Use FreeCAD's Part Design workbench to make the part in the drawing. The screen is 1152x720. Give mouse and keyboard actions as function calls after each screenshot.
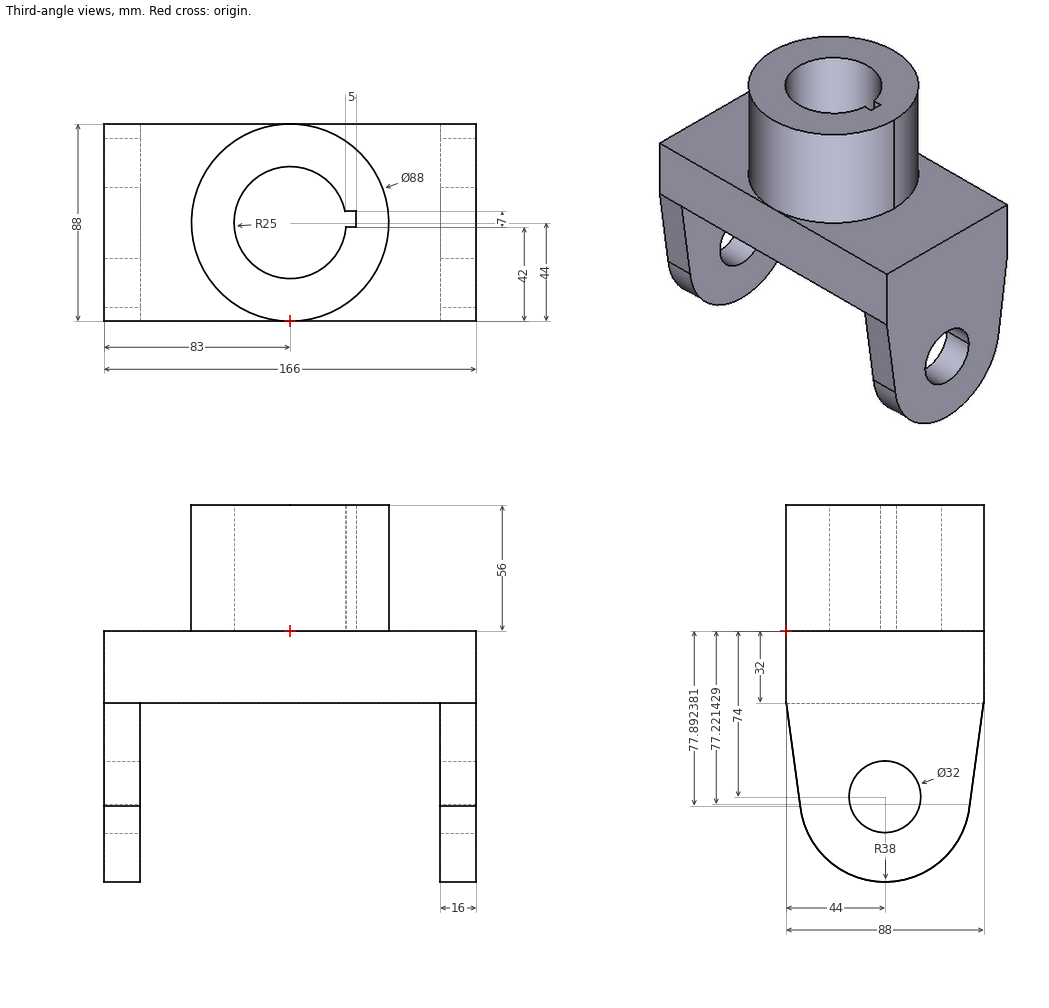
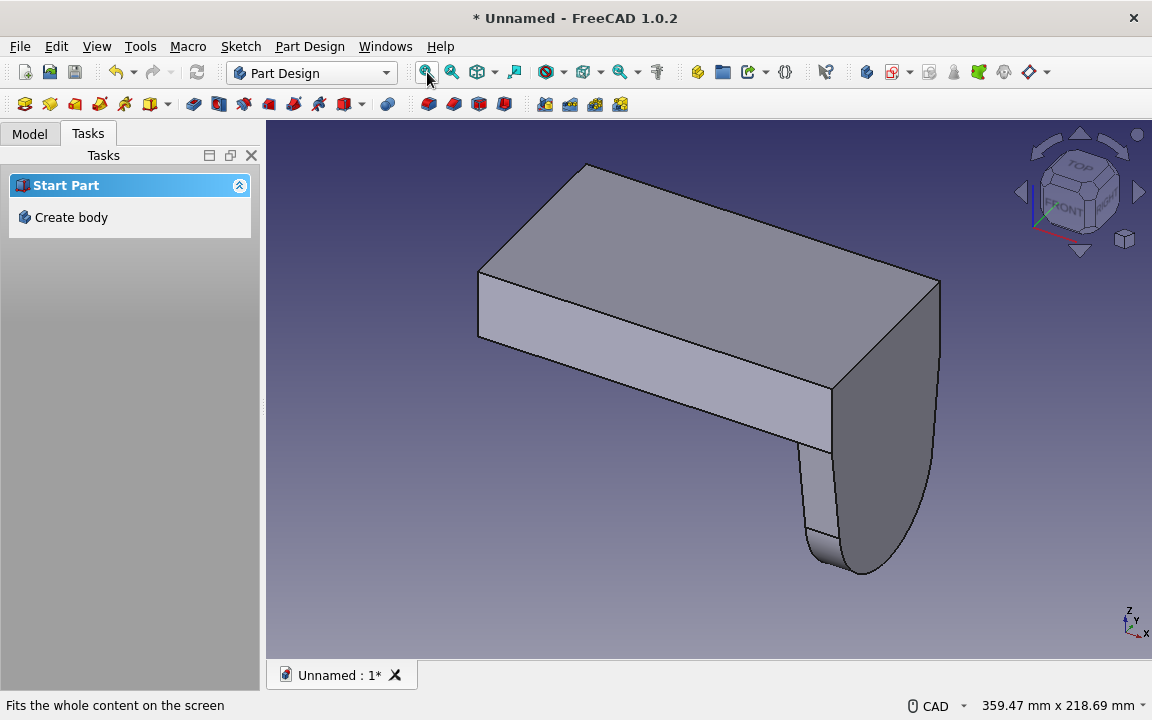
click(30, 134)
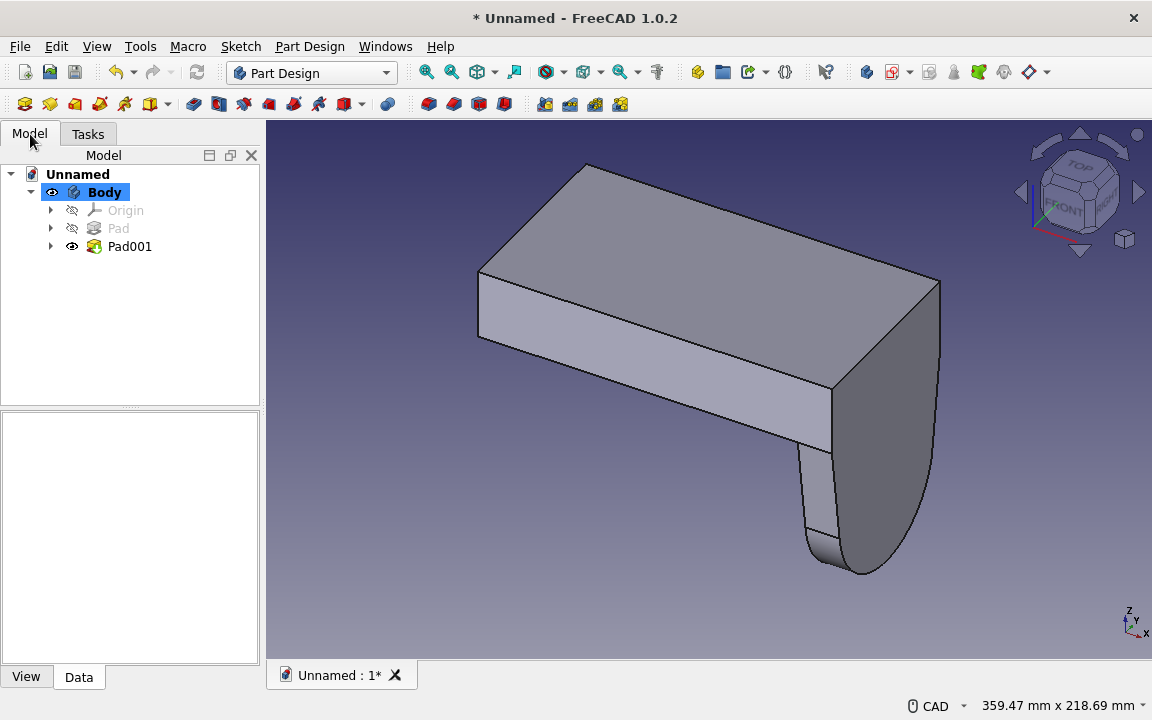
click(117, 246)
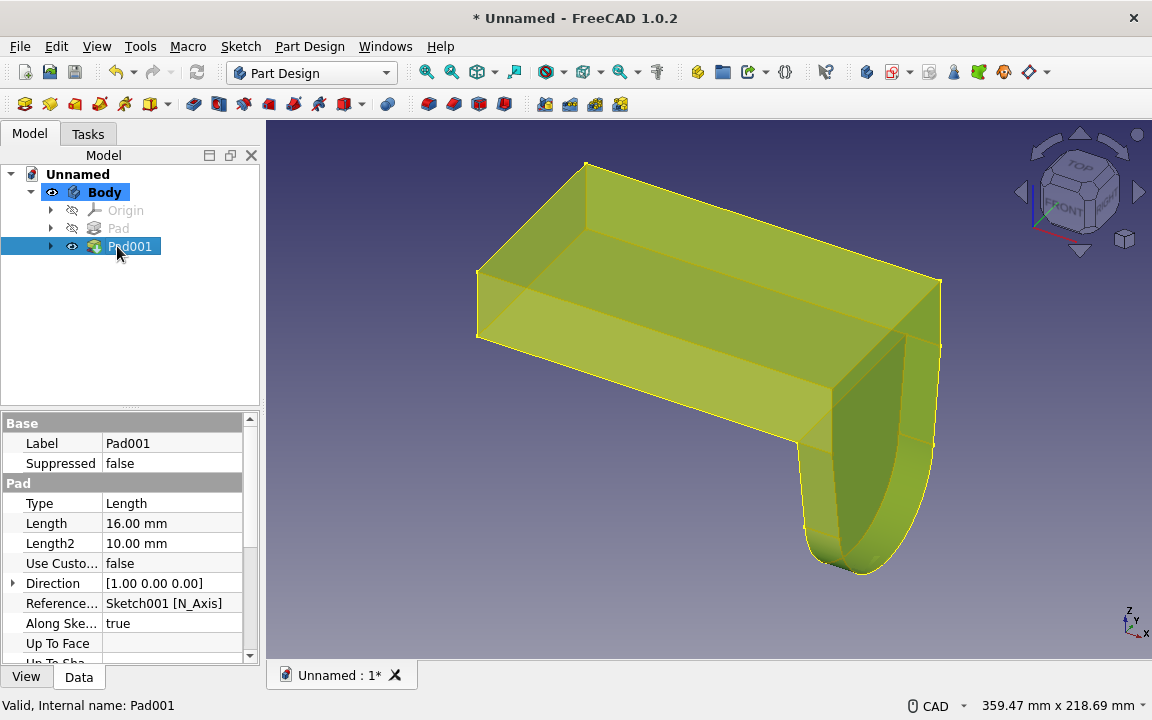
click(545, 104)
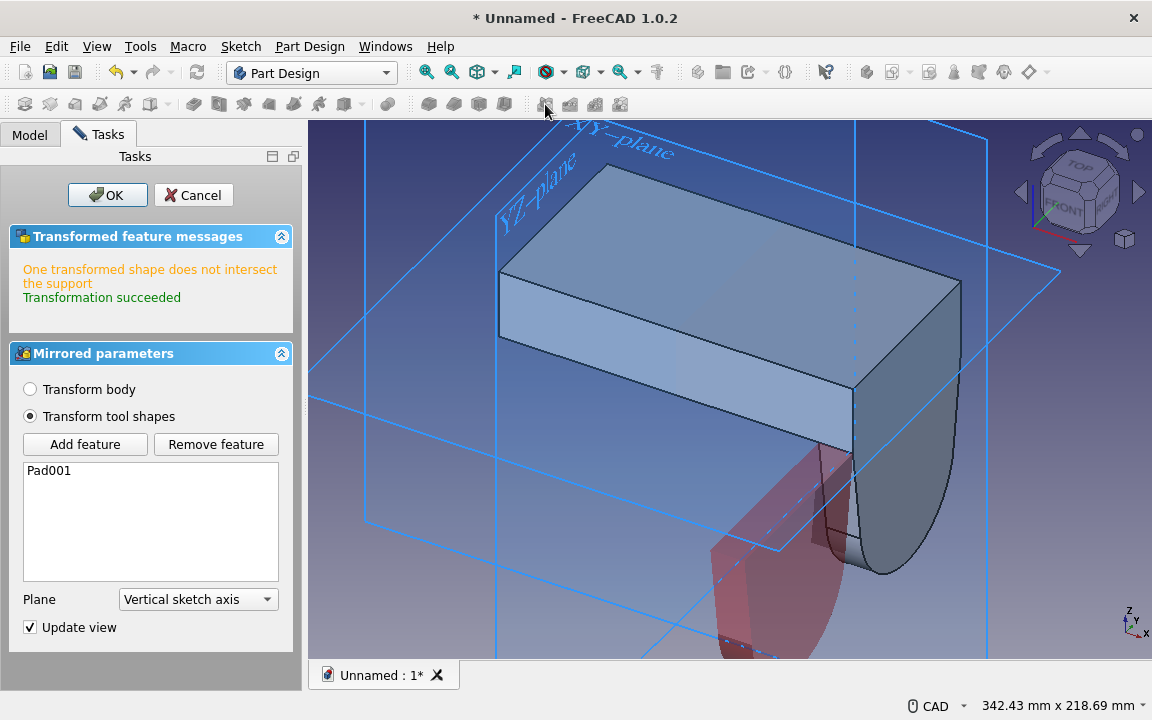
click(199, 600)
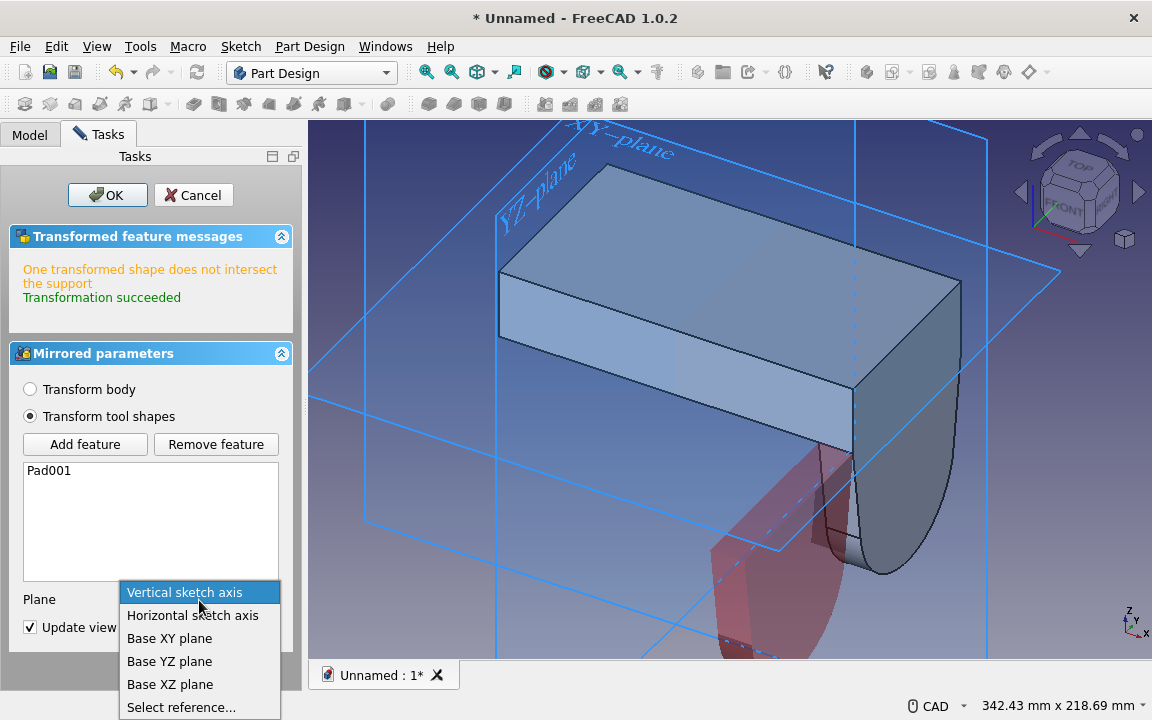
click(198, 662)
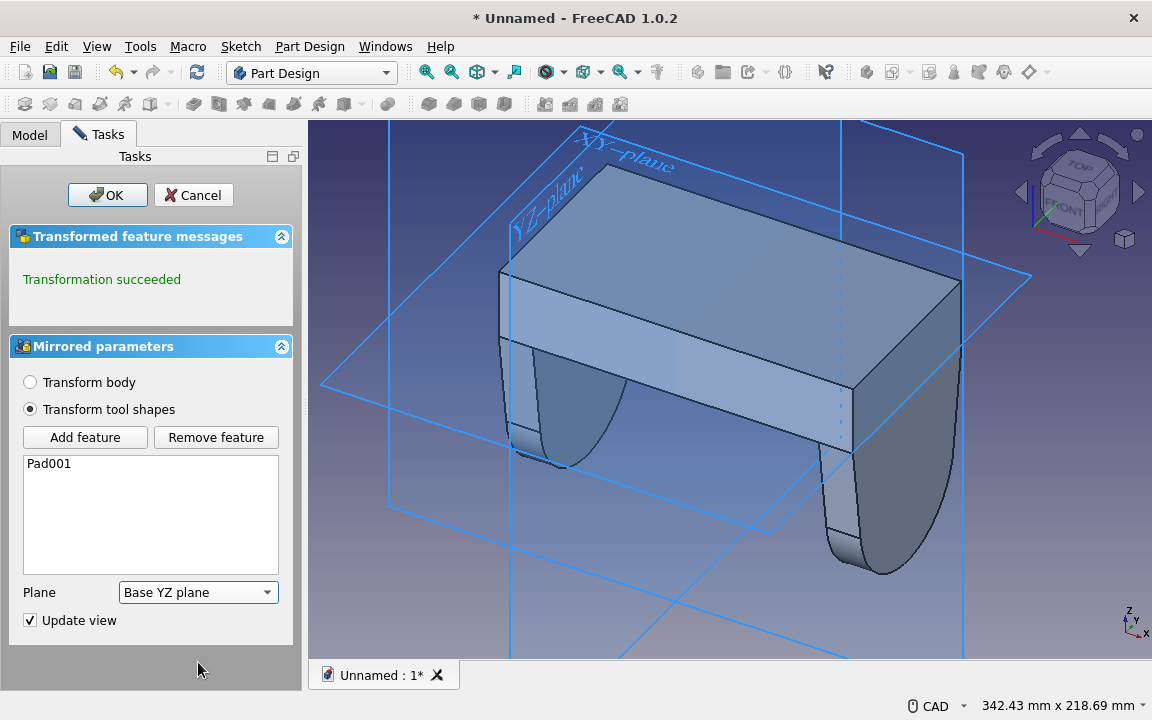
click(108, 195)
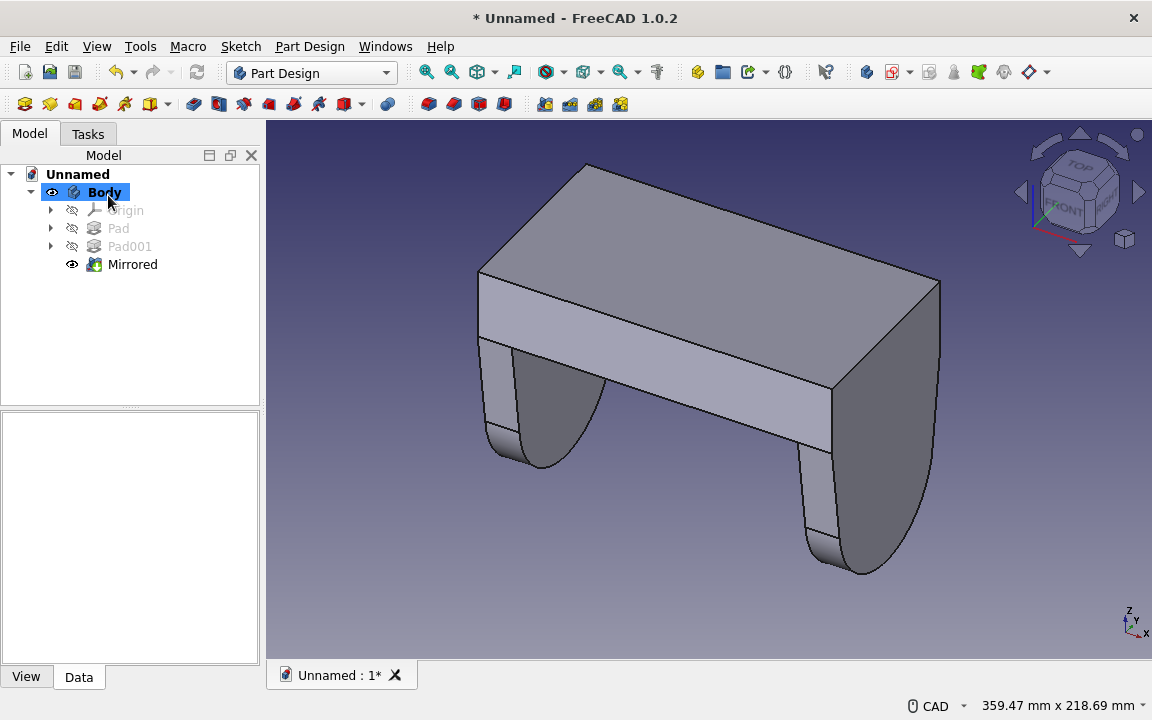
click(760, 292)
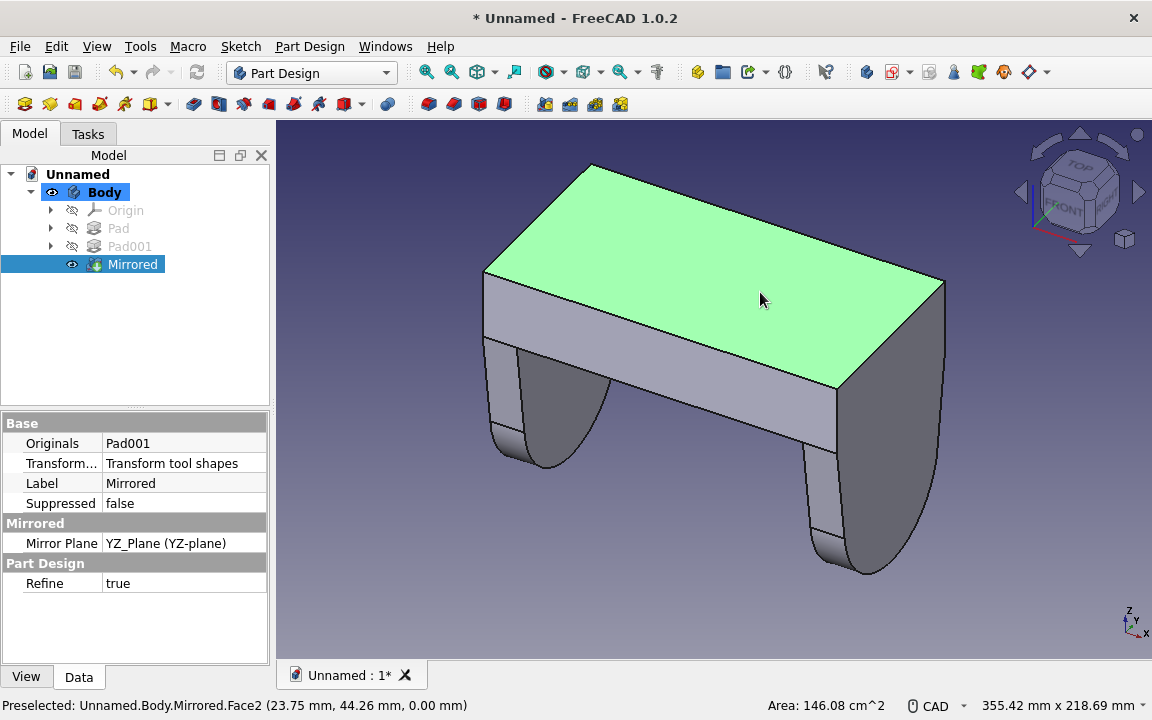
click(892, 72)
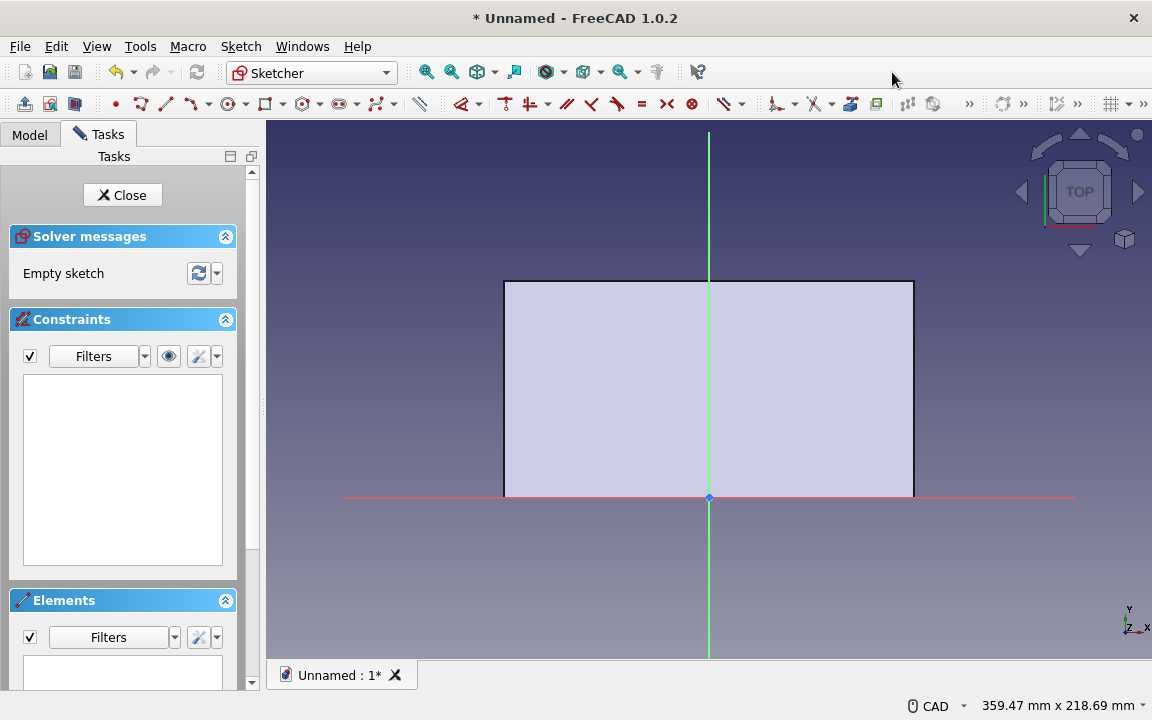
scroll(848, 390, up, 2)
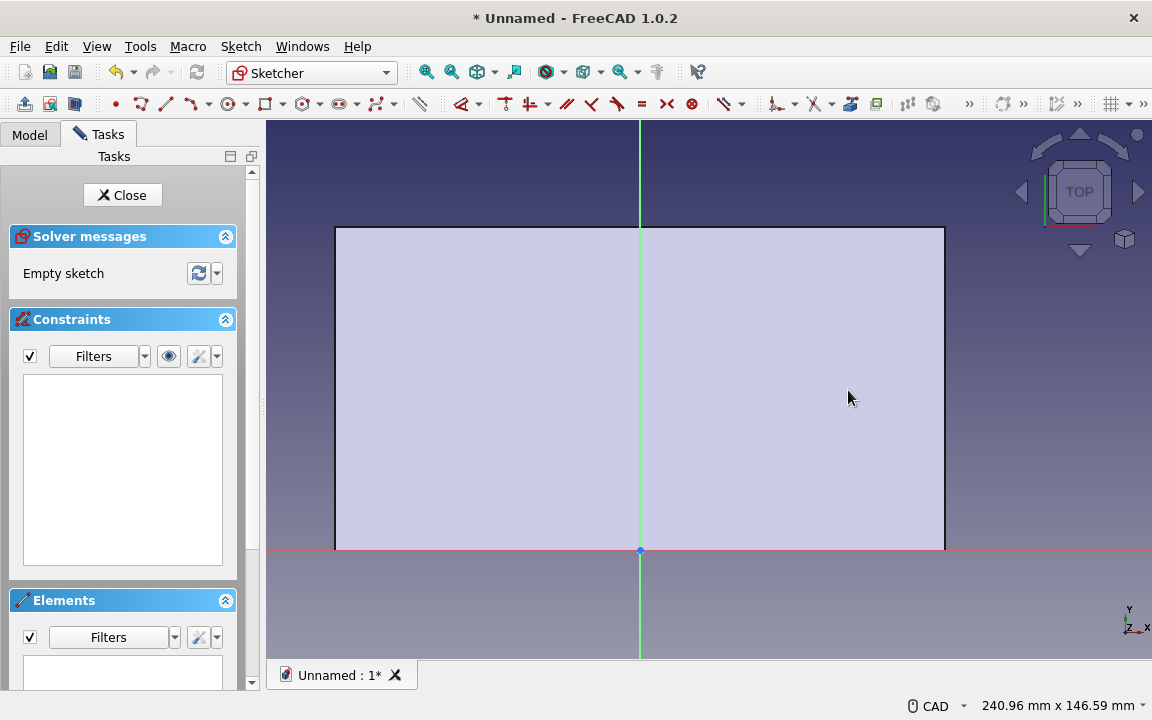
click(228, 104)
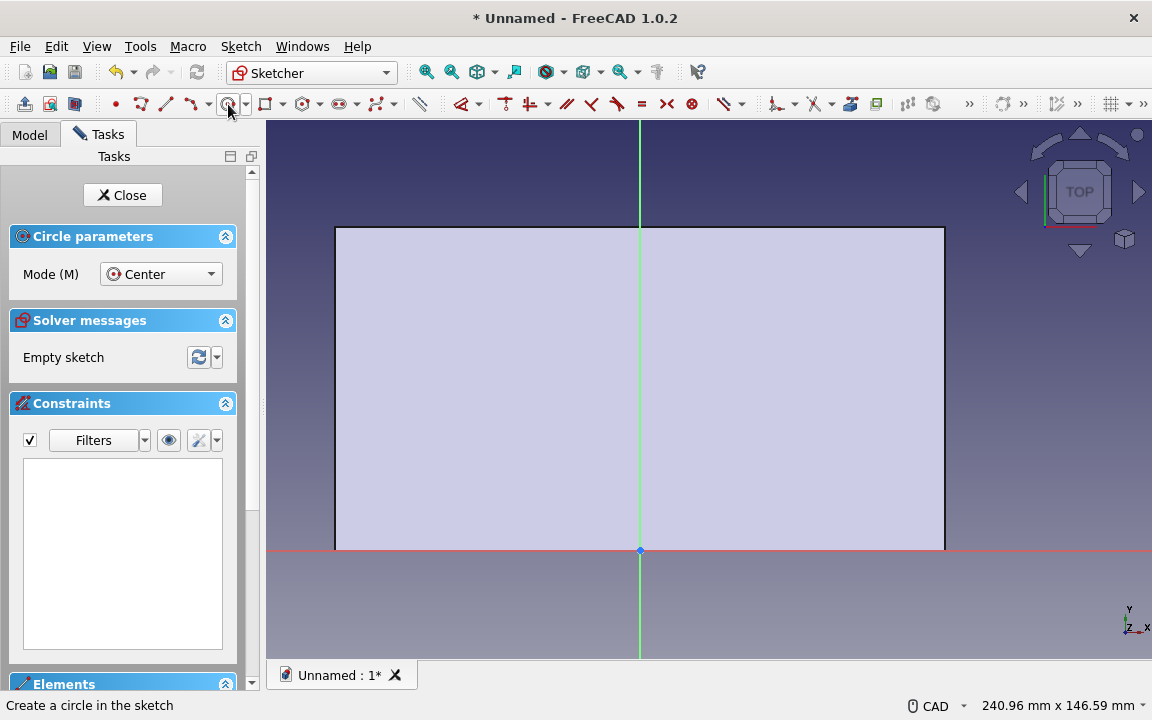
click(640, 389)
move(755, 275)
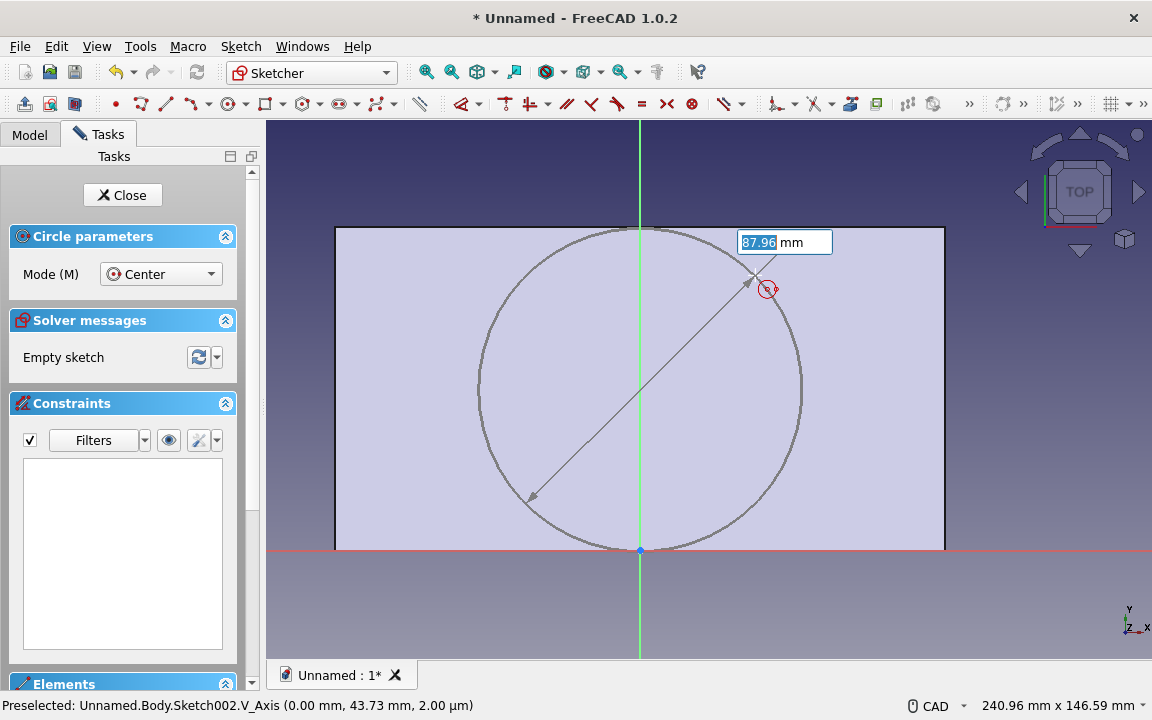
text(88)
key(Return)
key(Escape)